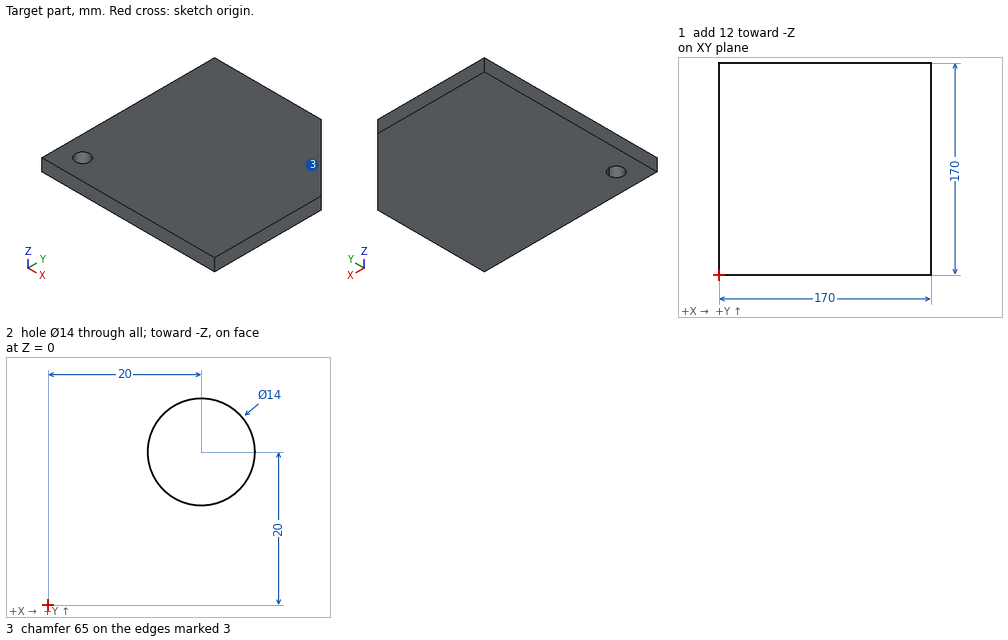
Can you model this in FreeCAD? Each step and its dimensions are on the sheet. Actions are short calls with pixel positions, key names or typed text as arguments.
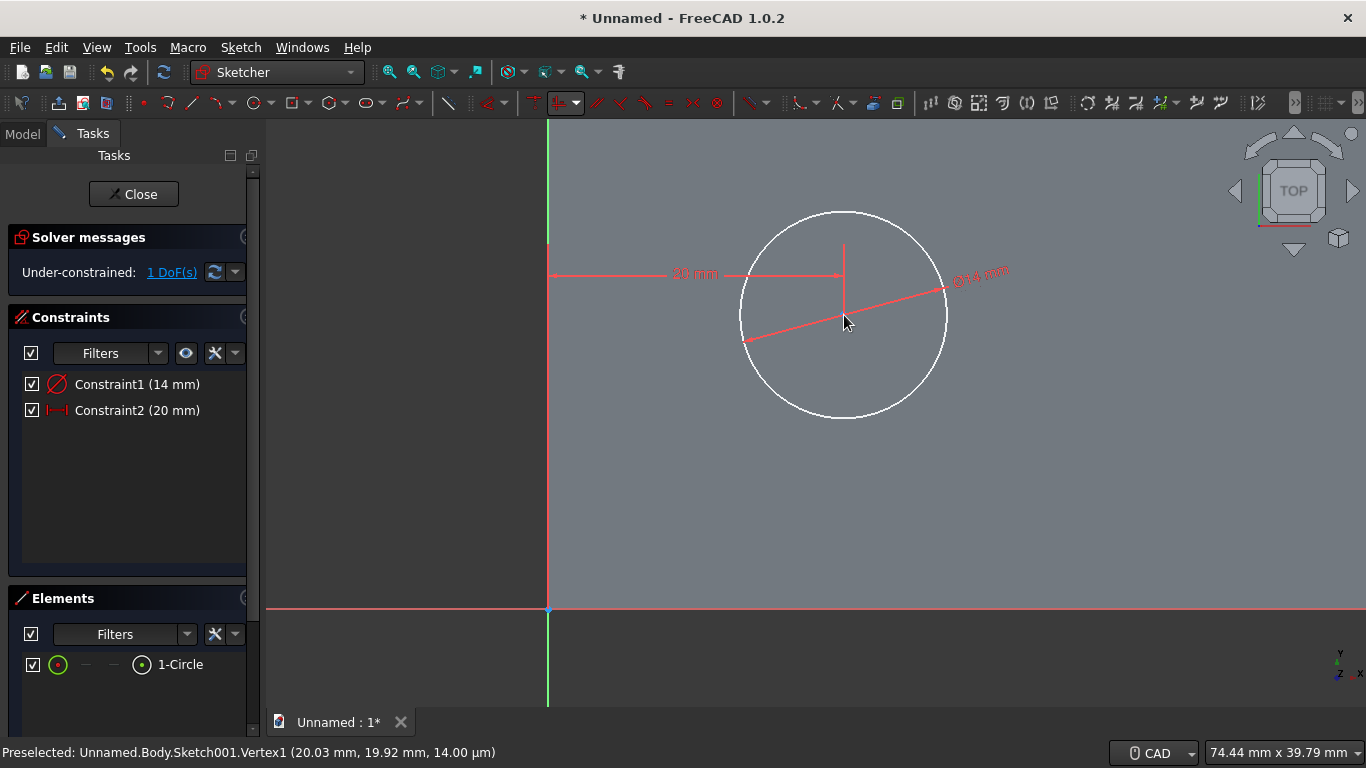
click(844, 315)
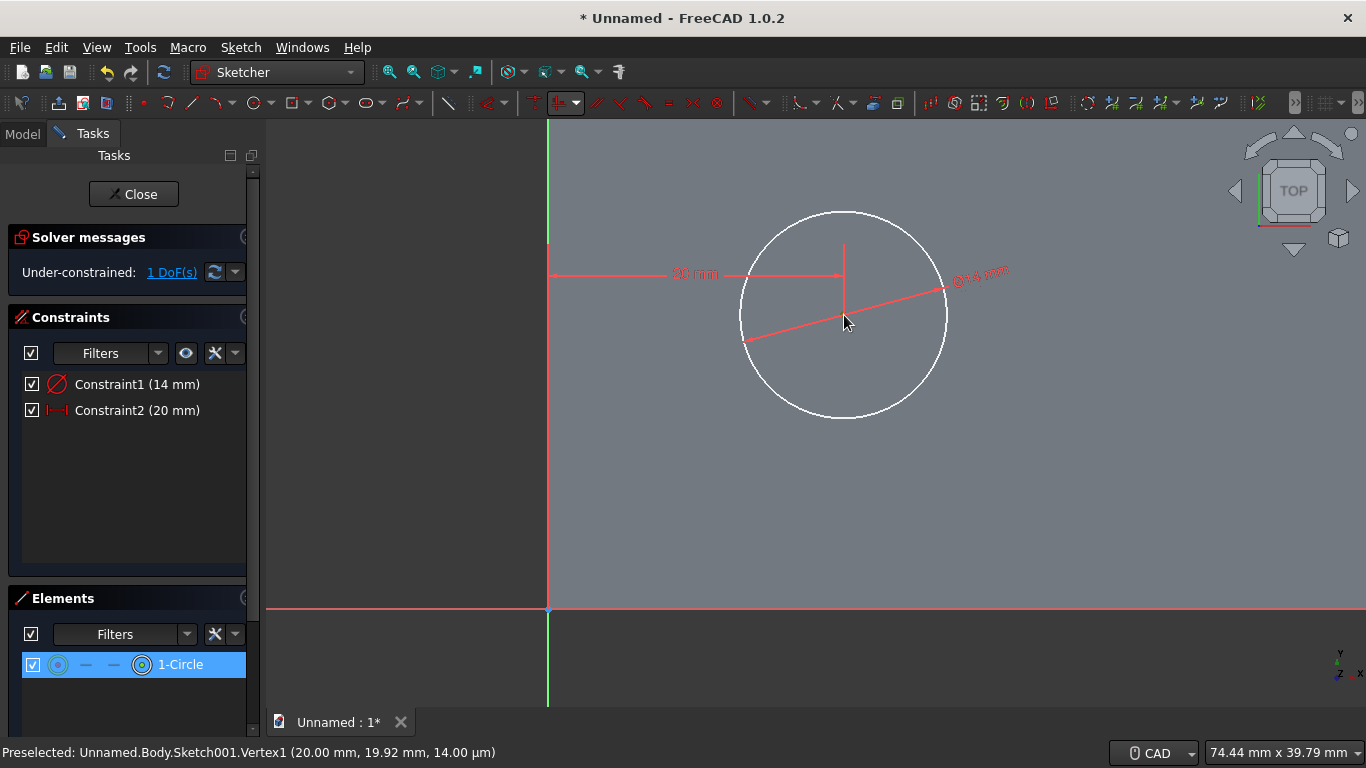
click(506, 104)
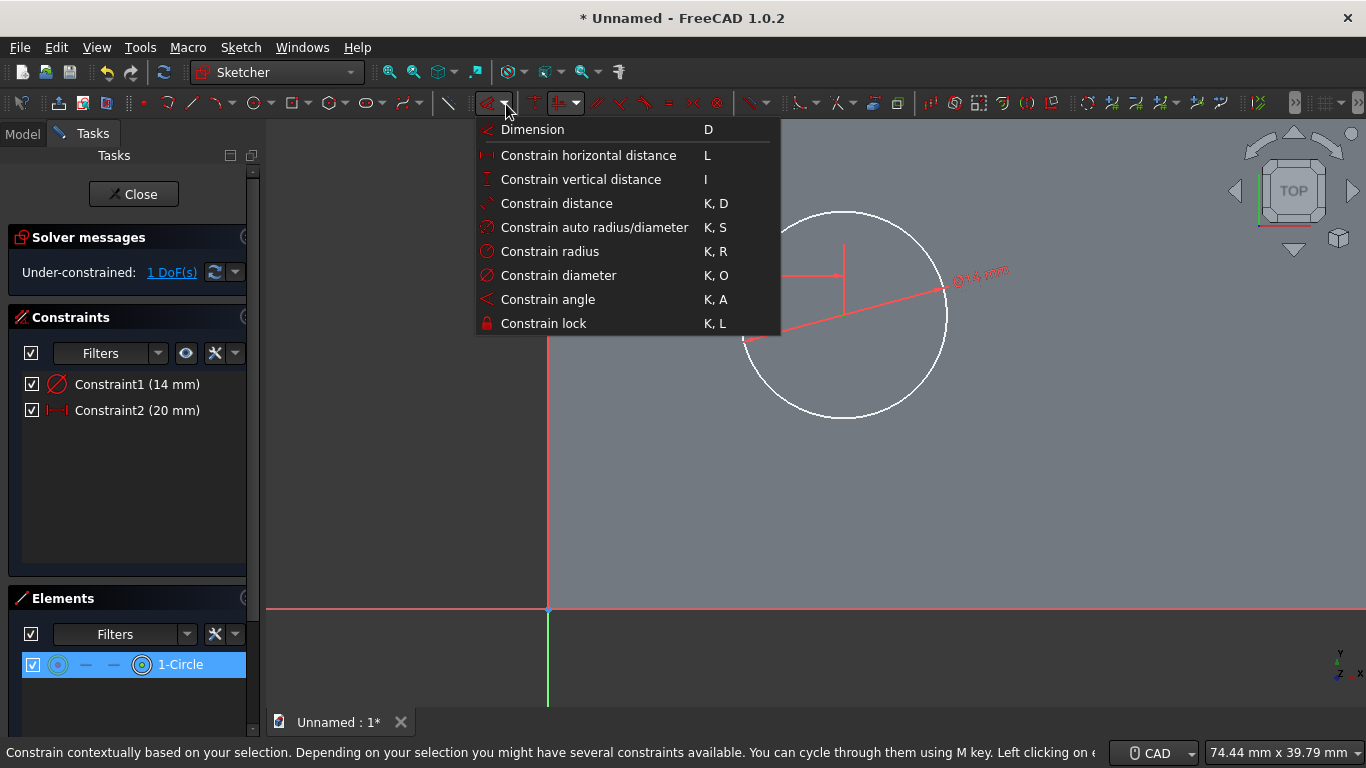
click(628, 179)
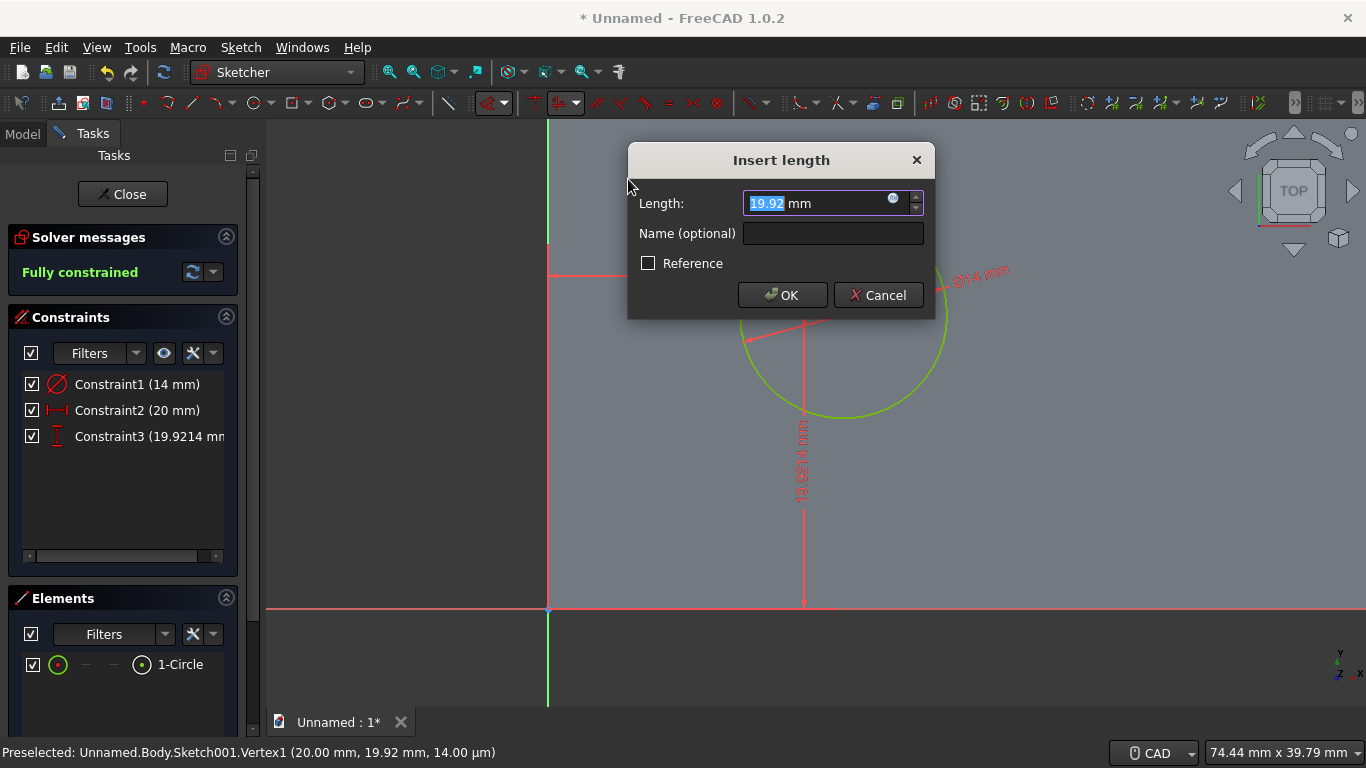
text(20)
key(Return)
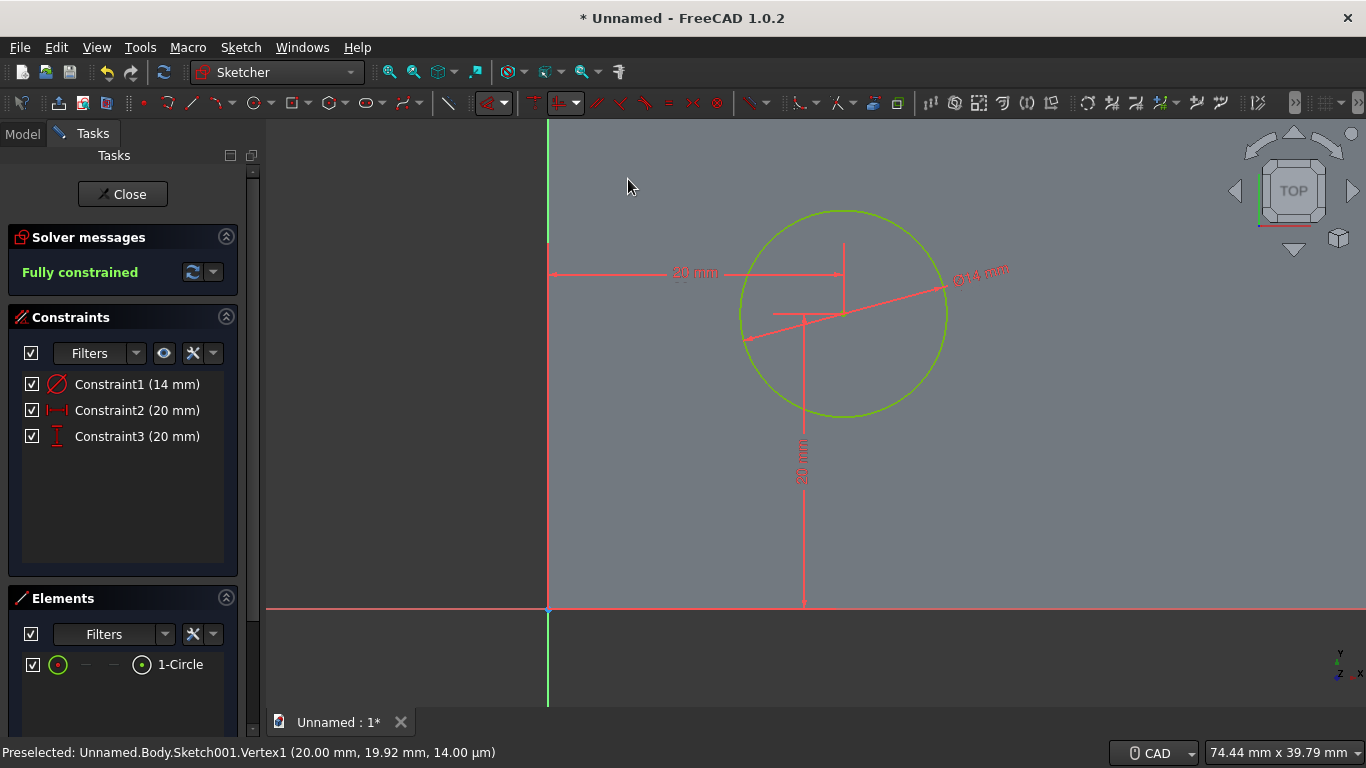
click(123, 194)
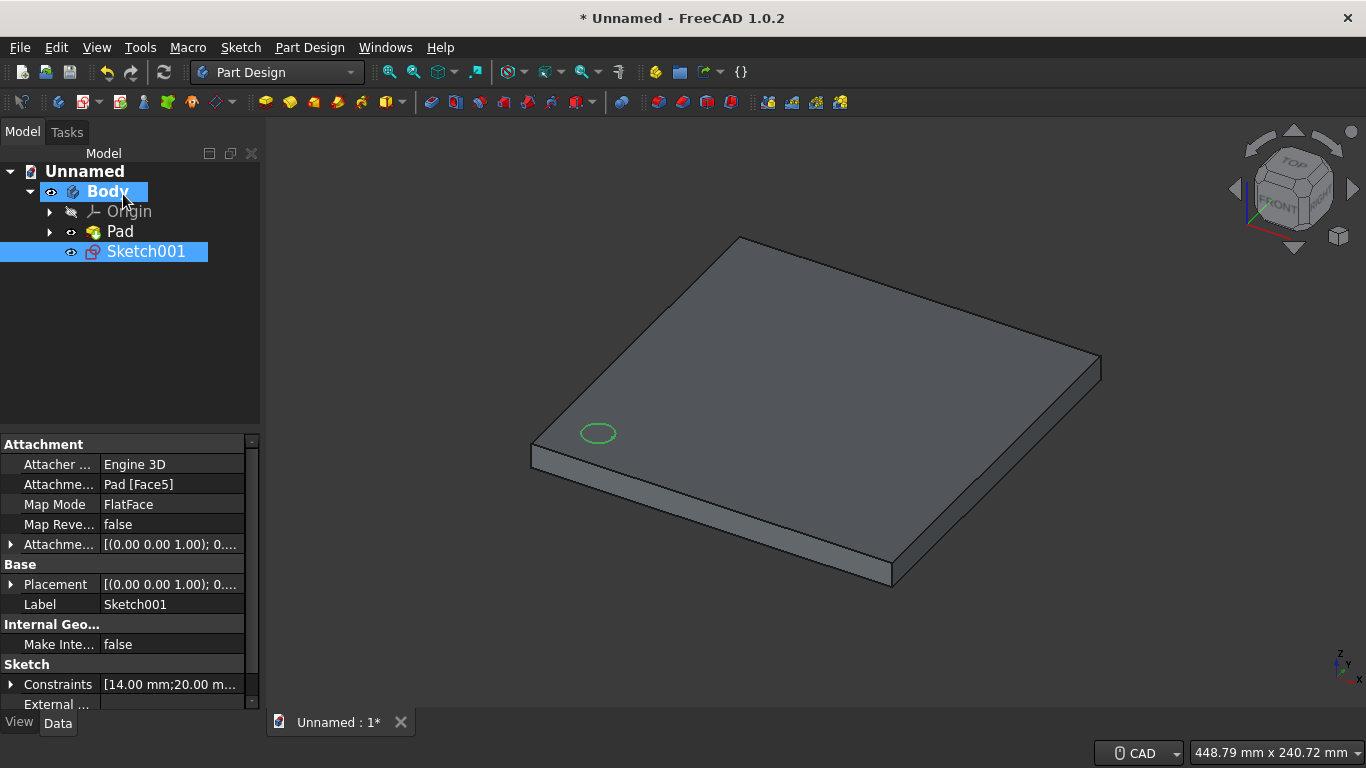
click(456, 102)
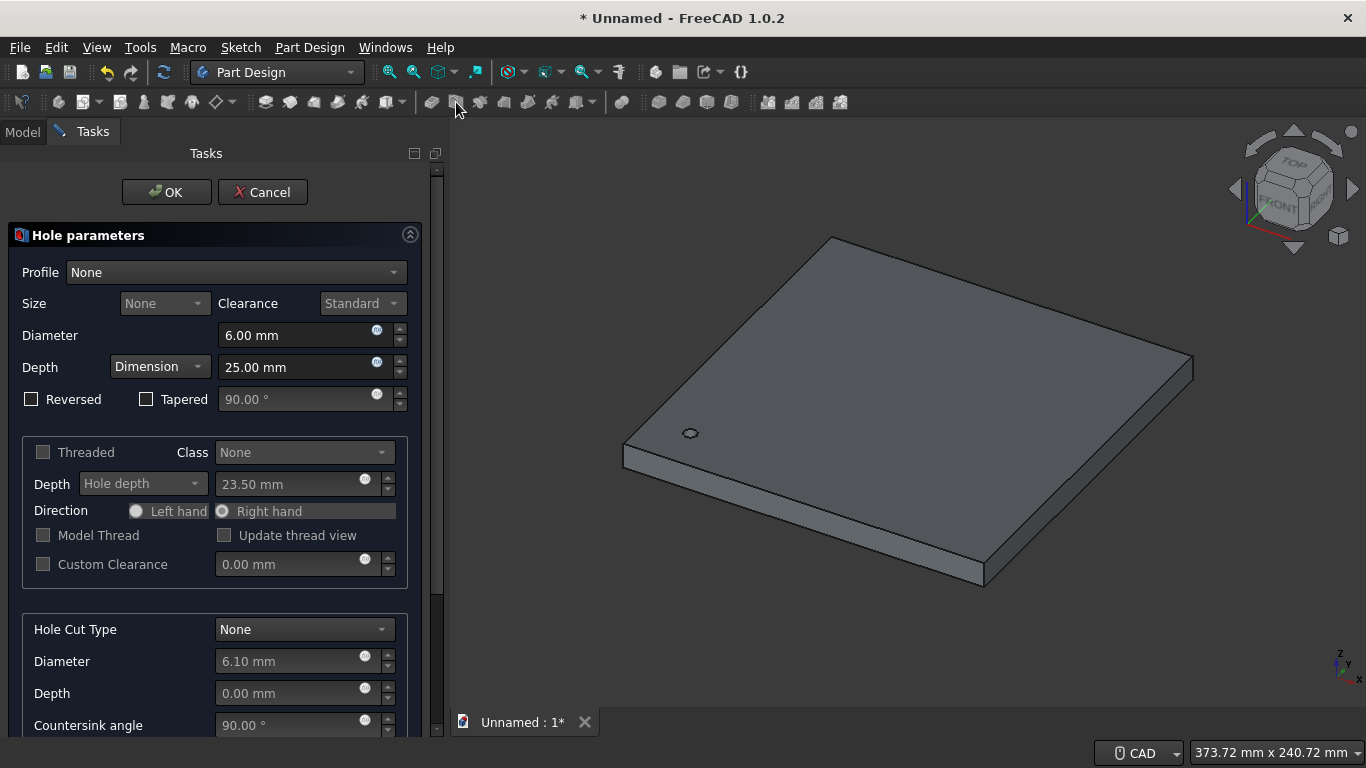
triple_click(305, 335)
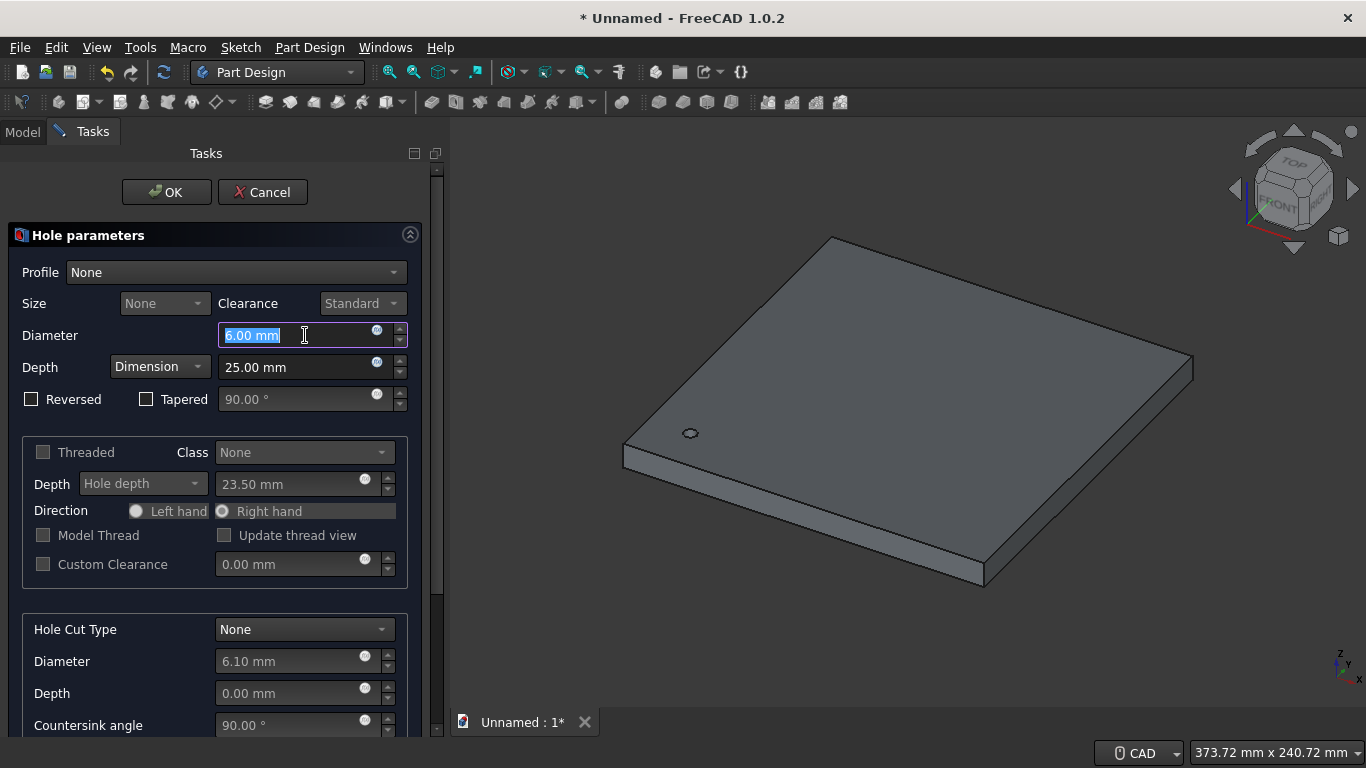
text(14)
key(Tab)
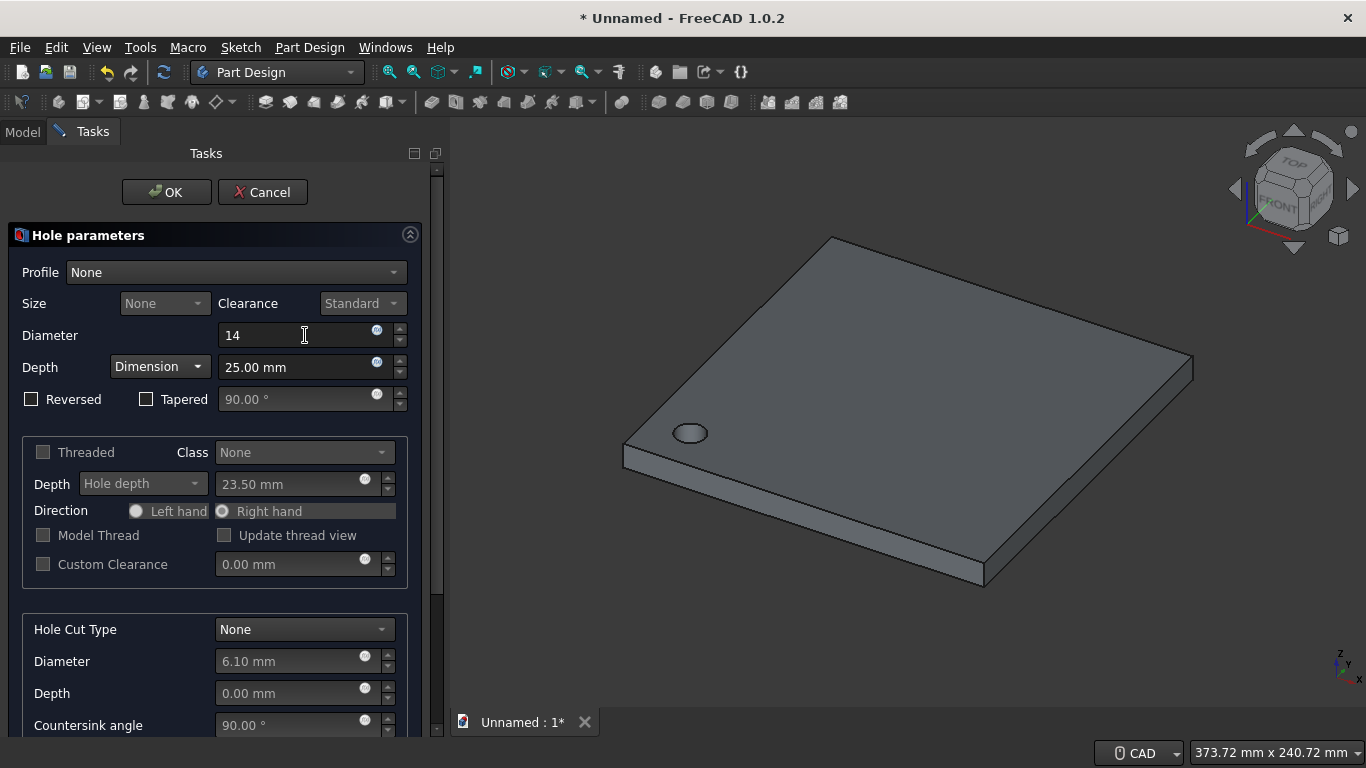
click(161, 366)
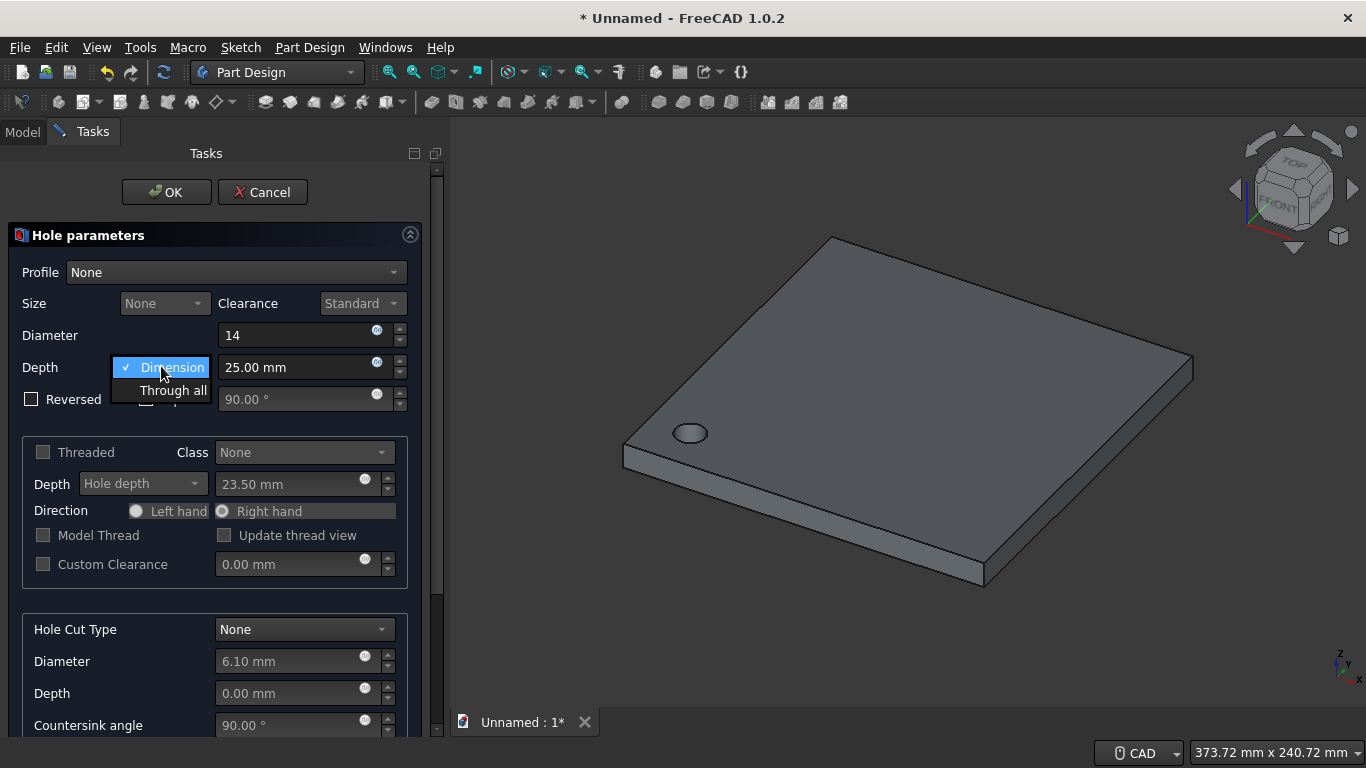
click(160, 390)